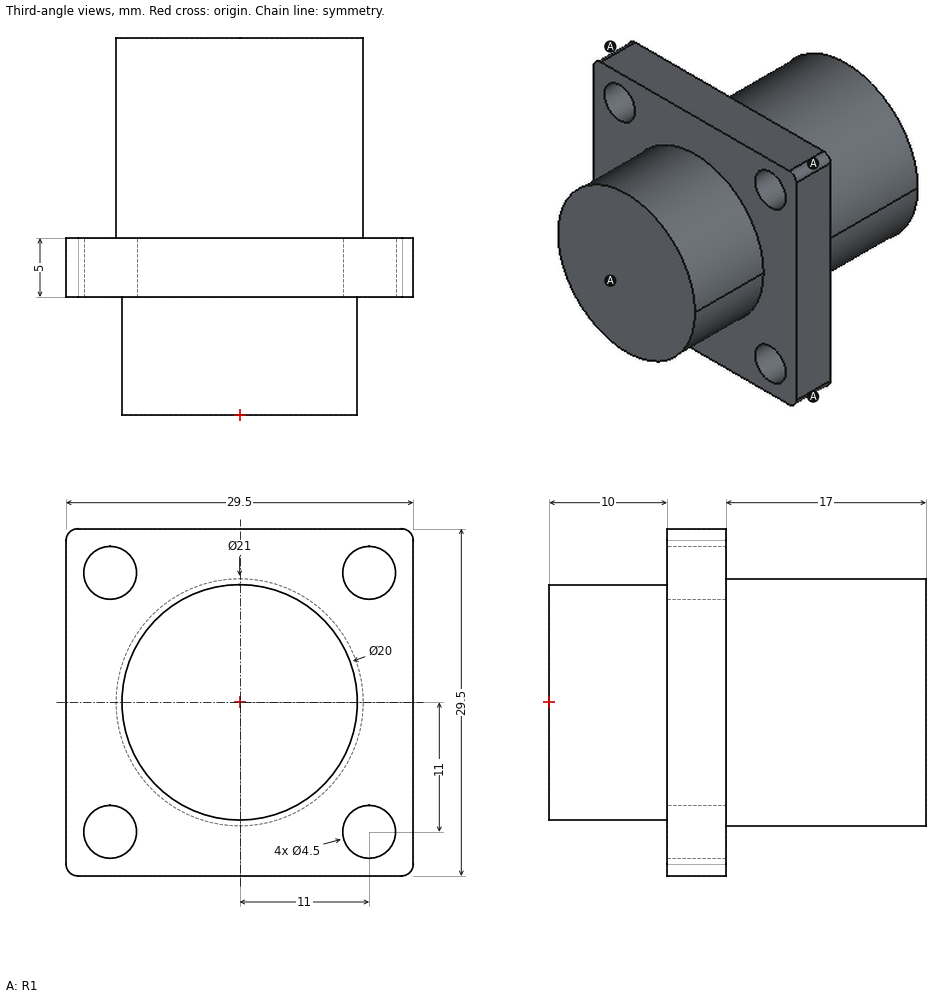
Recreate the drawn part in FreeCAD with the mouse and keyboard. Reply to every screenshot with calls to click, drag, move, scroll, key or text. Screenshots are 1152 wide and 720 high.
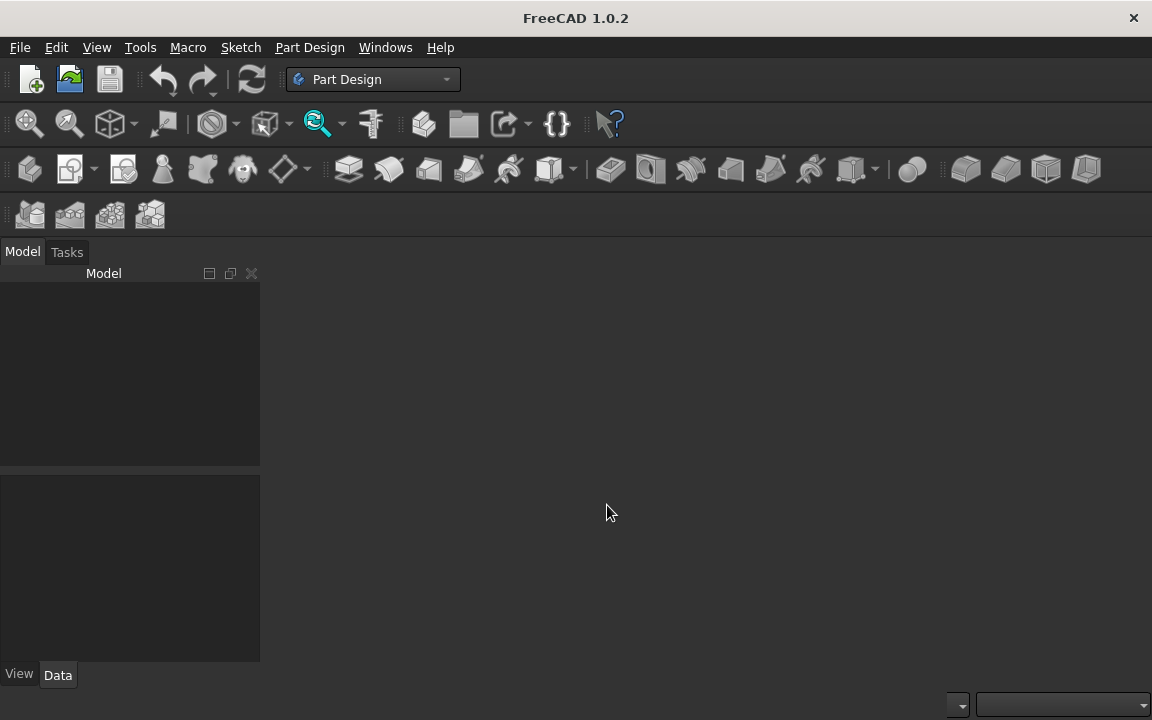
key(ctrl+n)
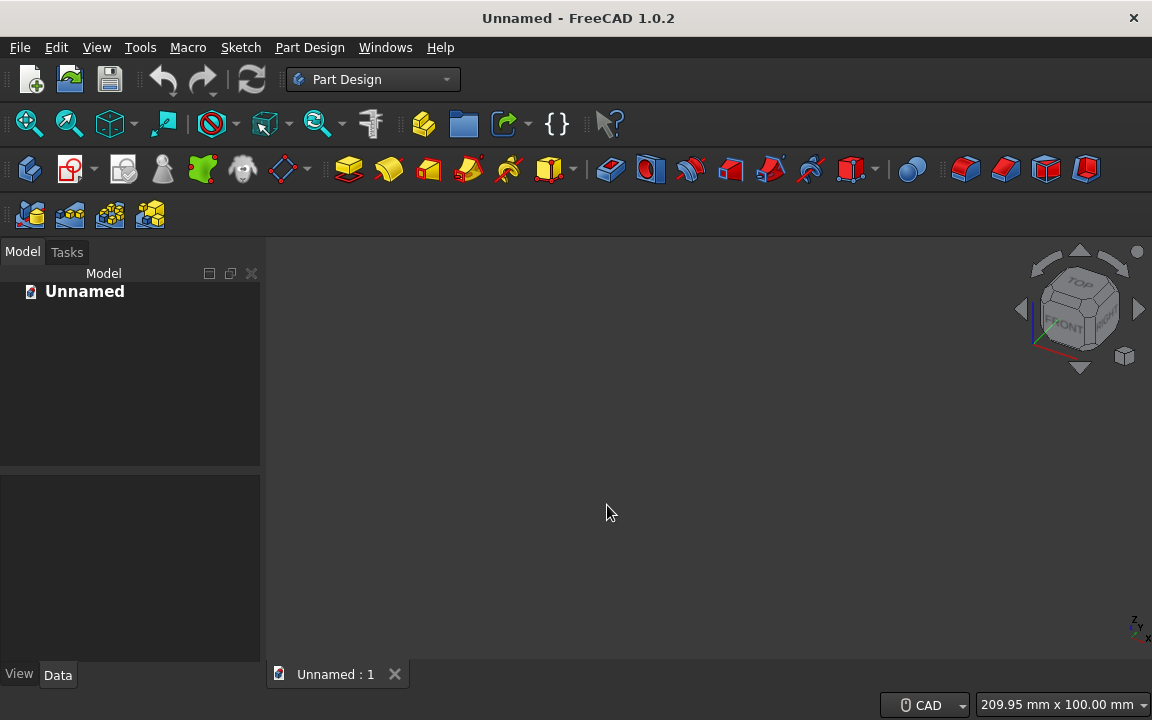
click(70, 170)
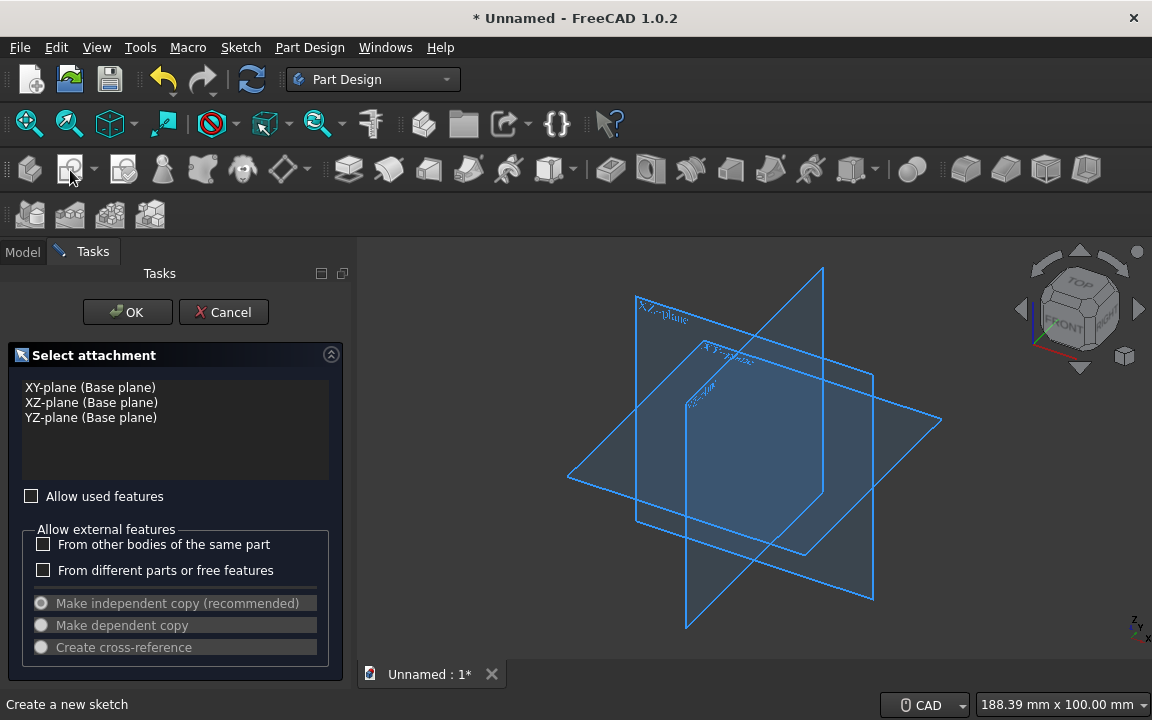
click(82, 402)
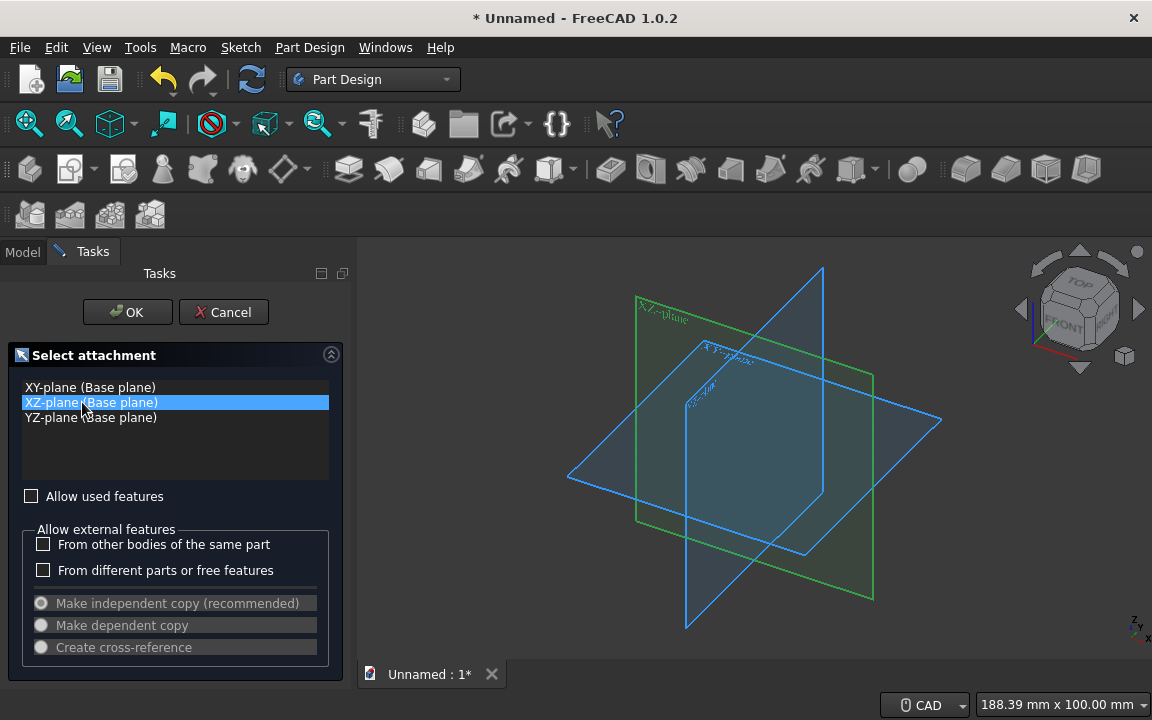
click(128, 312)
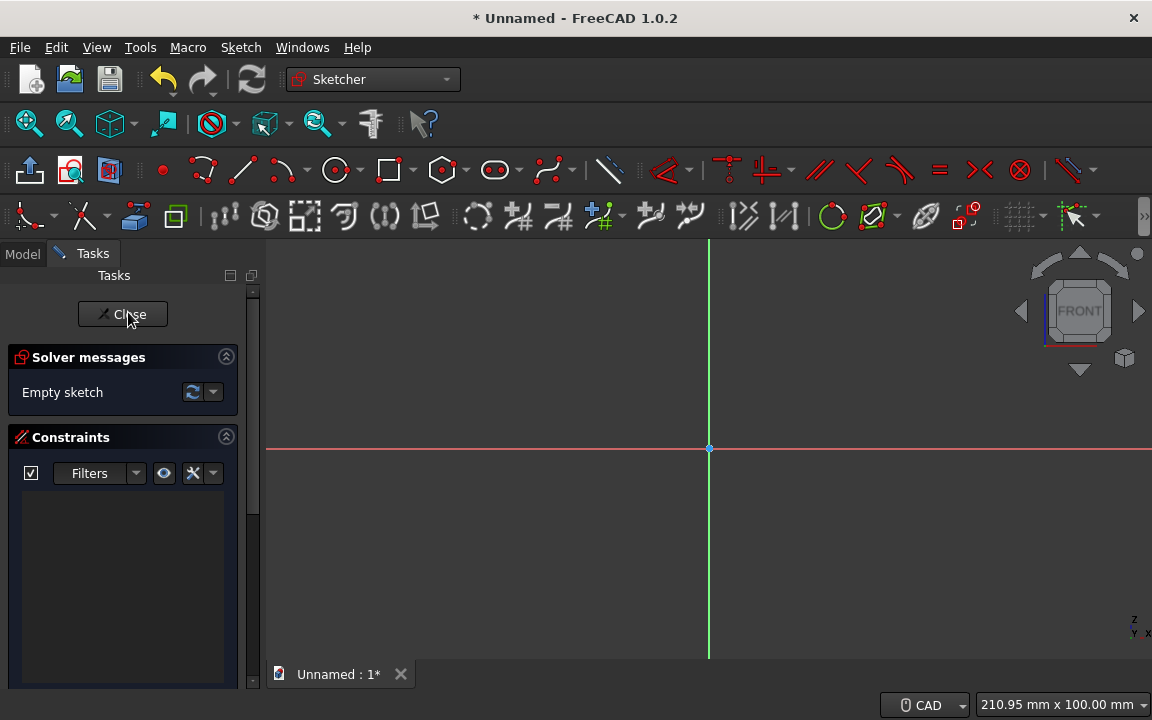
scroll(739, 449, up, 6)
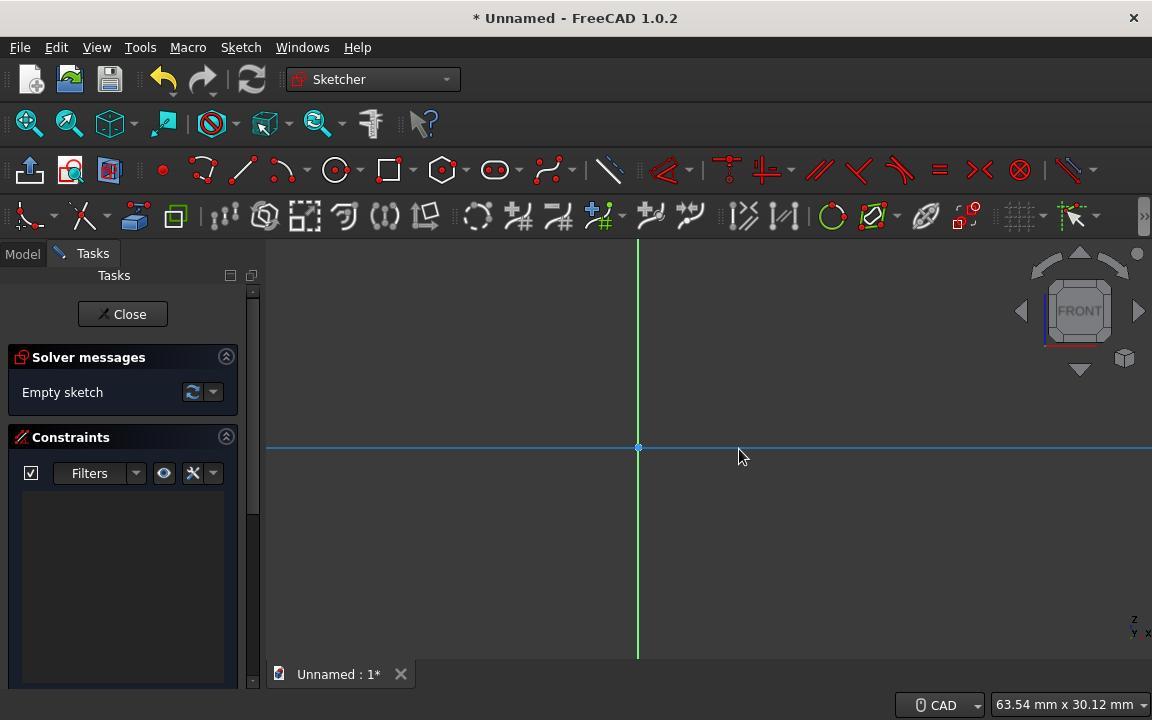
key(g)
key(c)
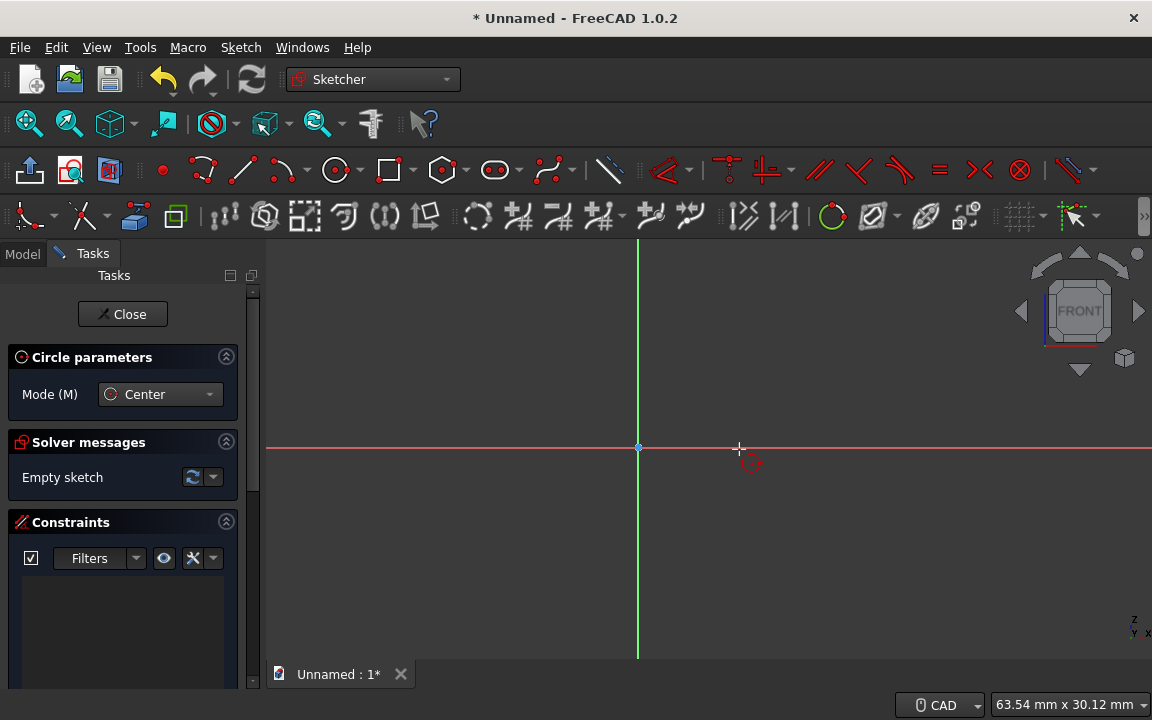
click(638, 448)
move(737, 349)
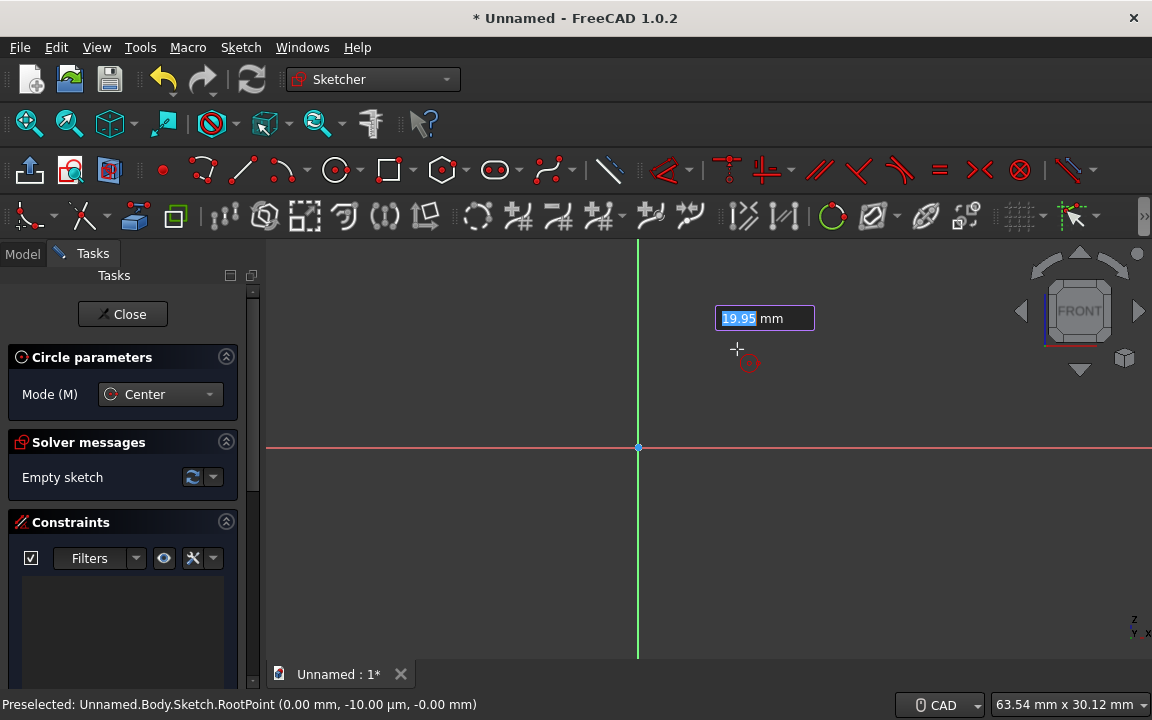
text(20)
key(Return)
key(Escape)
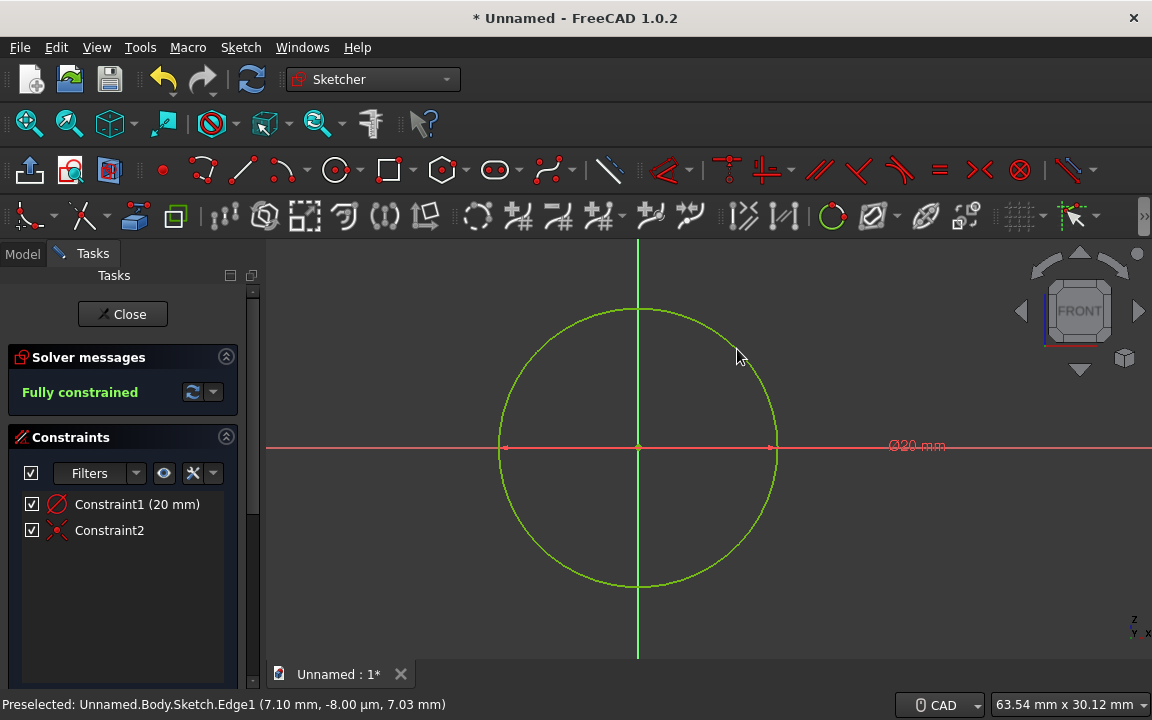
click(123, 314)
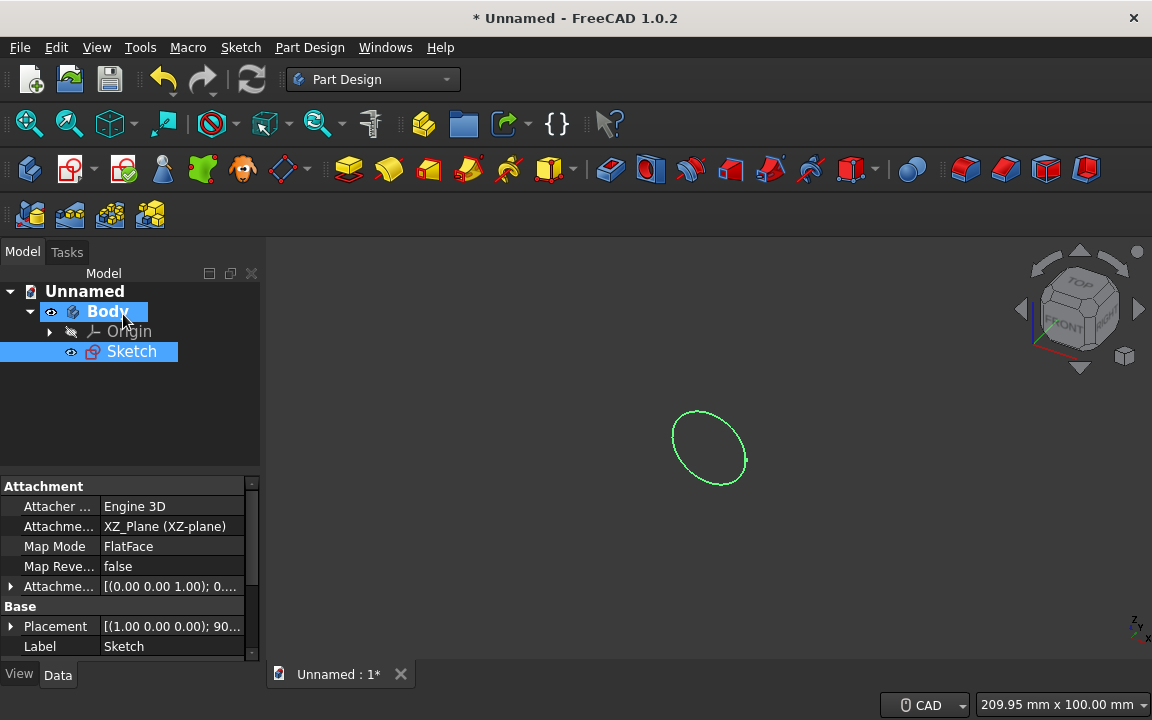
click(350, 170)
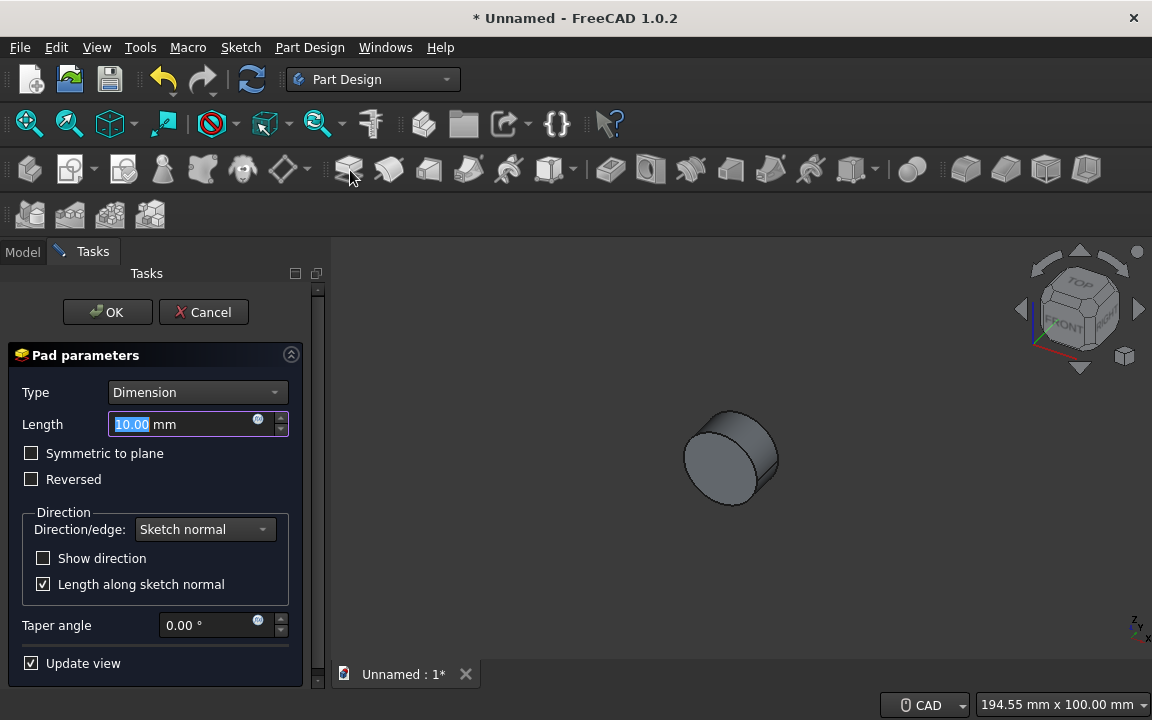
text(10)
key(Tab)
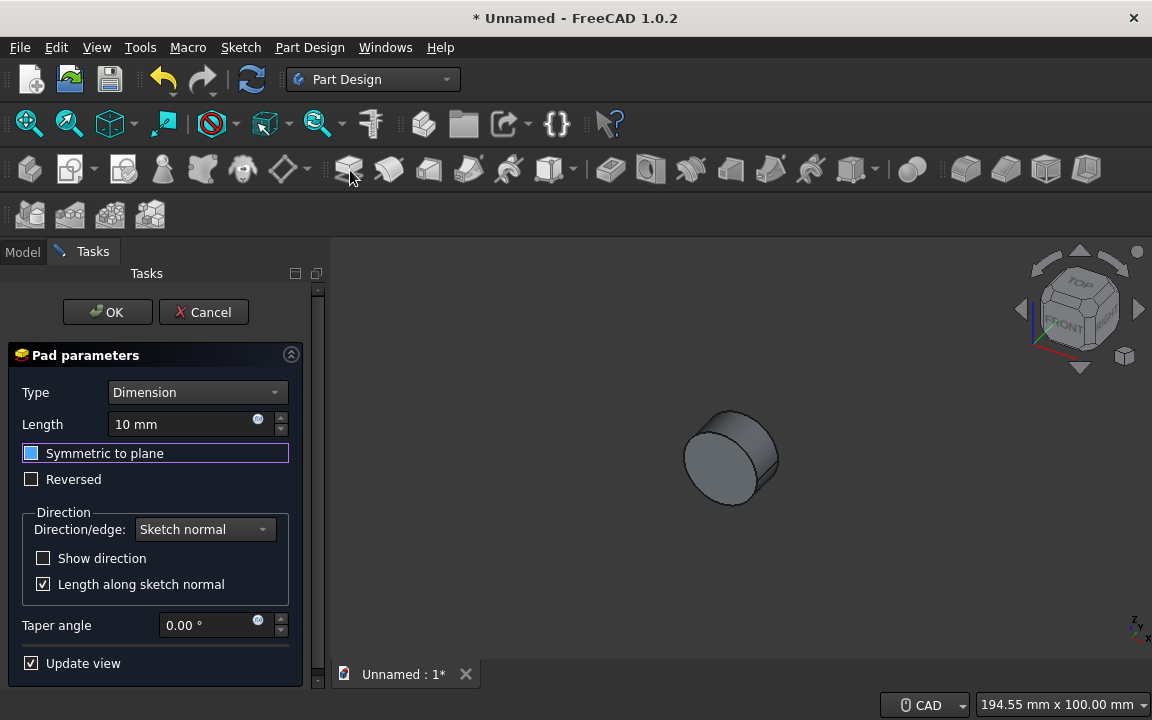
click(30, 479)